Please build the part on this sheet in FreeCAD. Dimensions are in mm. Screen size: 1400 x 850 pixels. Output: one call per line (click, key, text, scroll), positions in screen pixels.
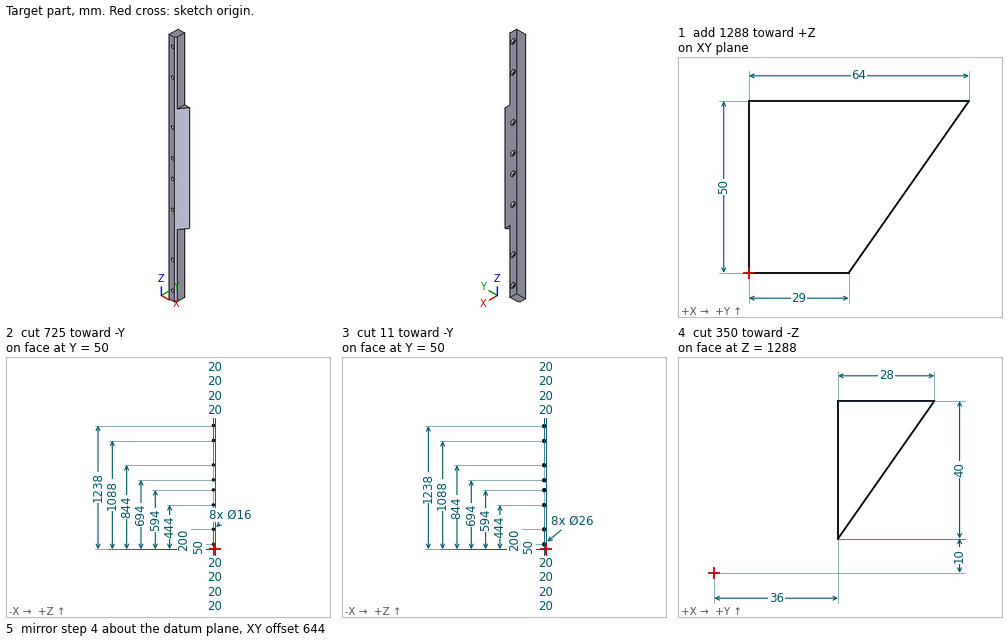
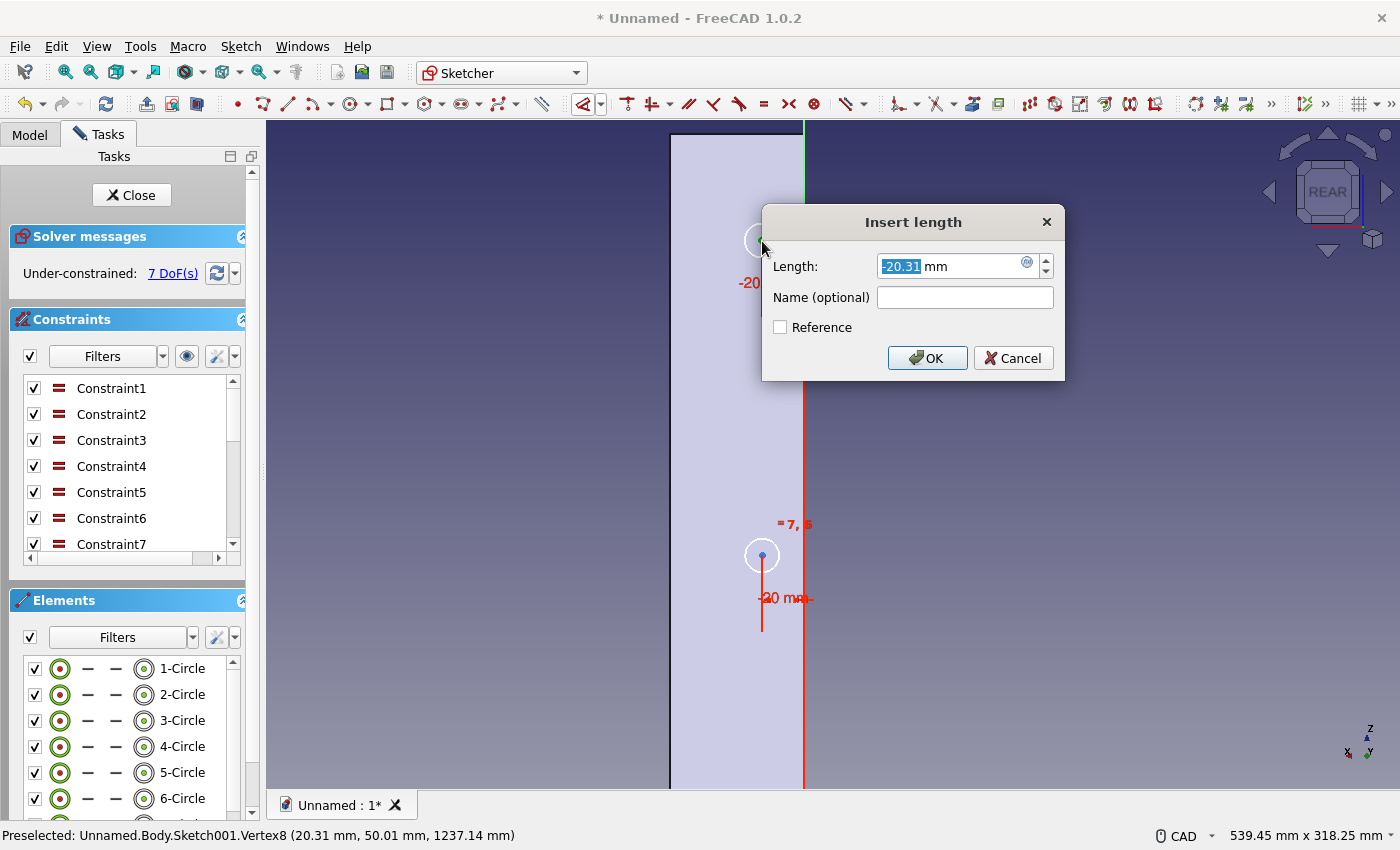
text(-20)
key(Return)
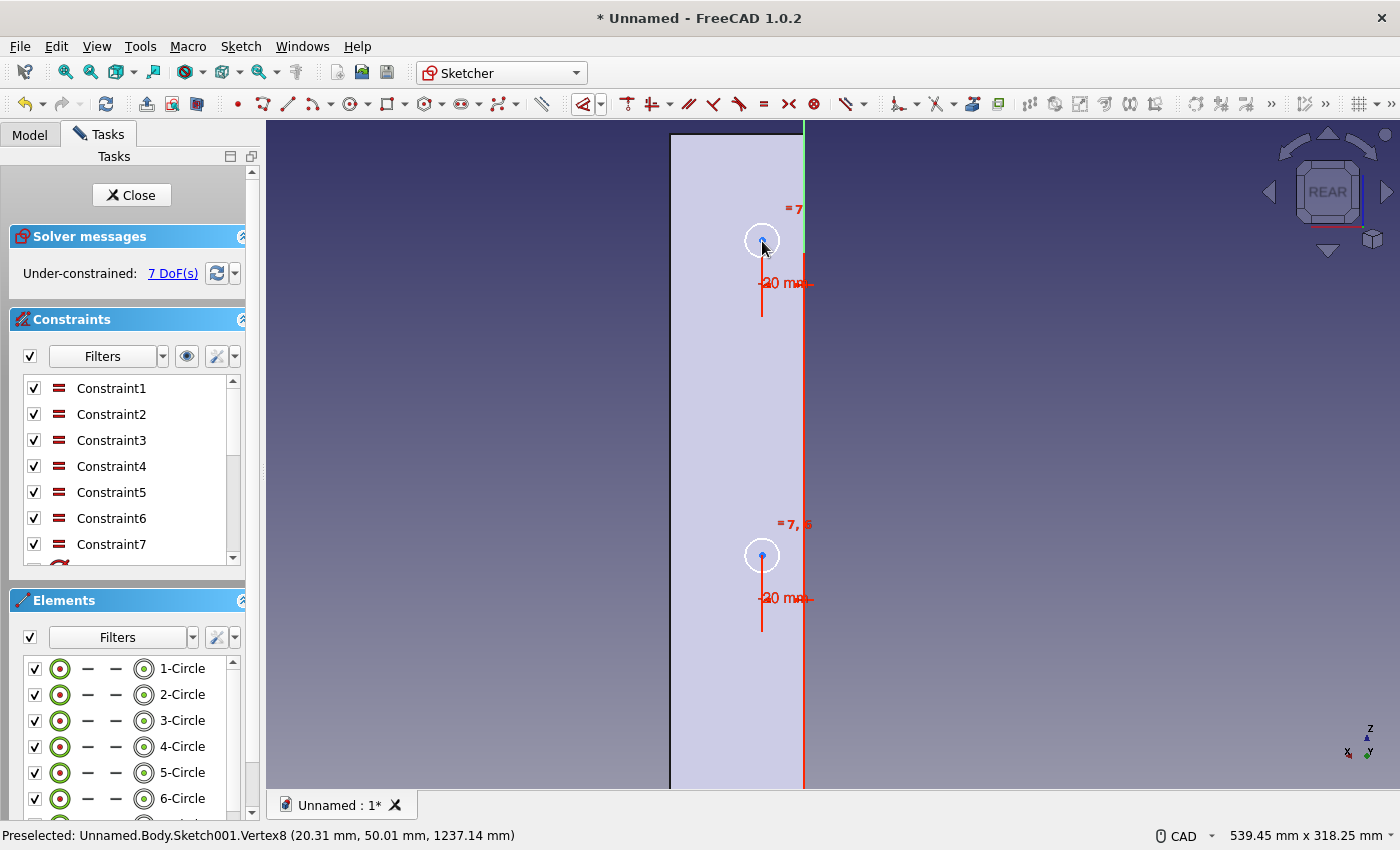
scroll(762, 241, down, 9)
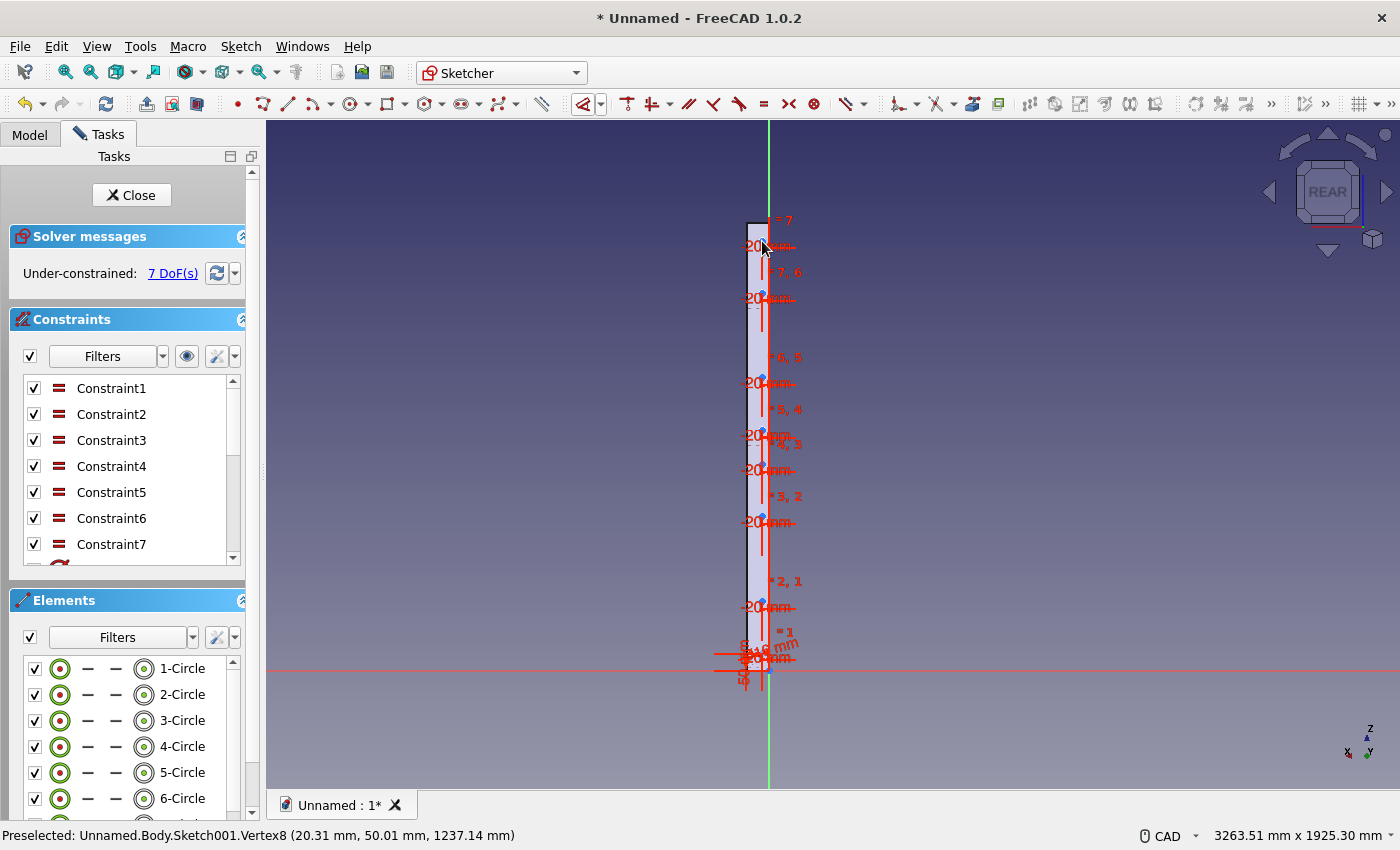
click(762, 602)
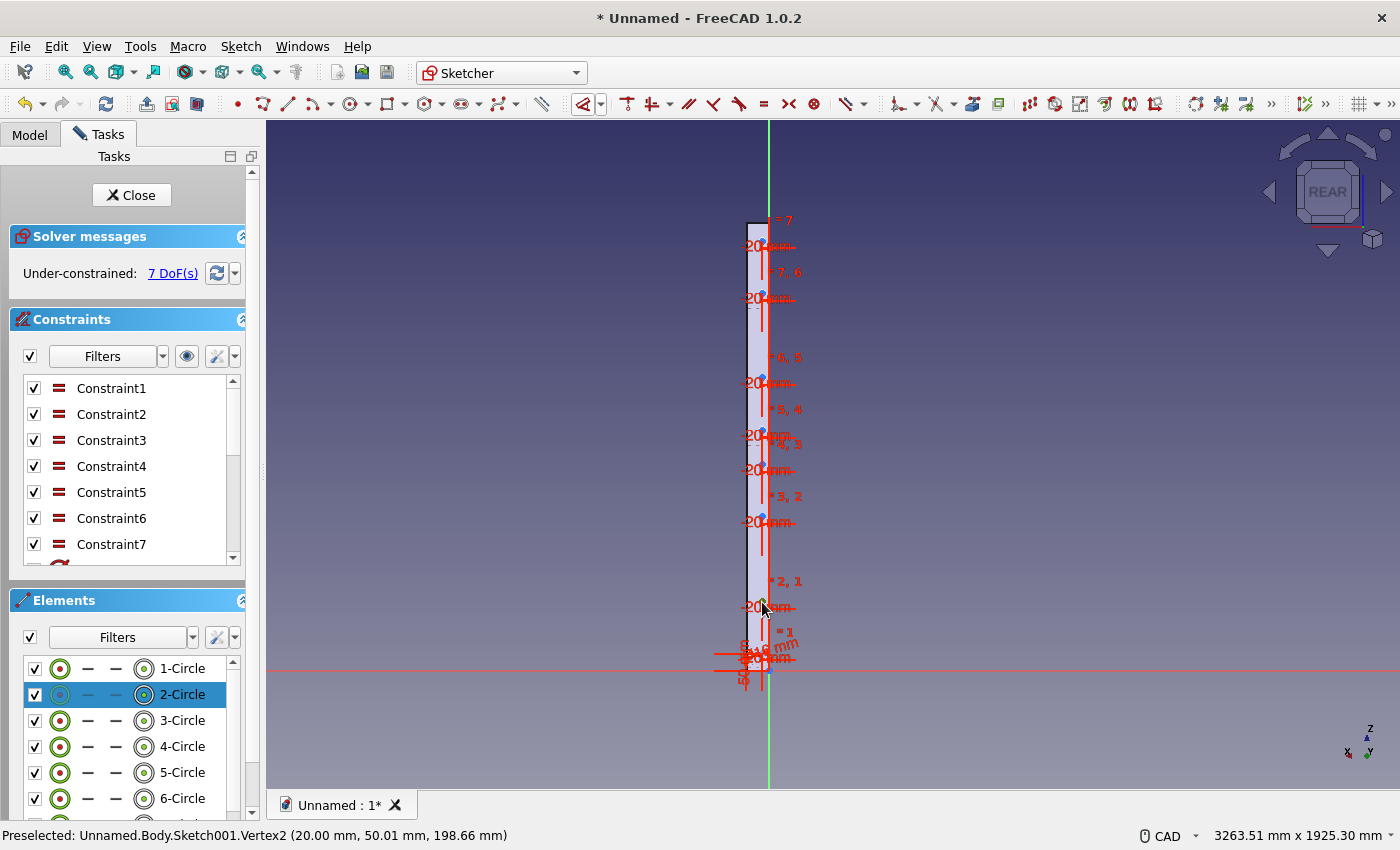
key(i)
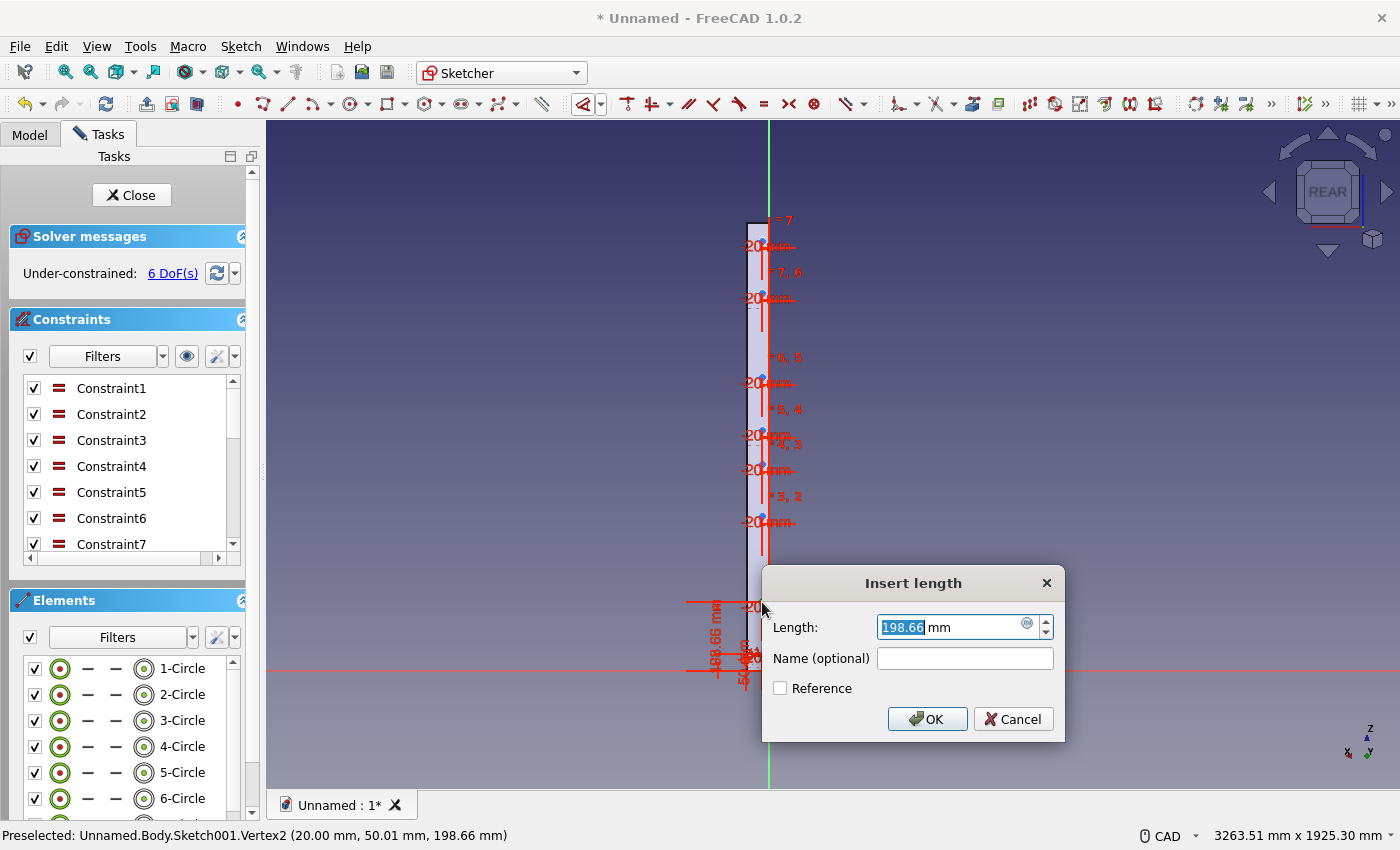
text(200)
key(Return)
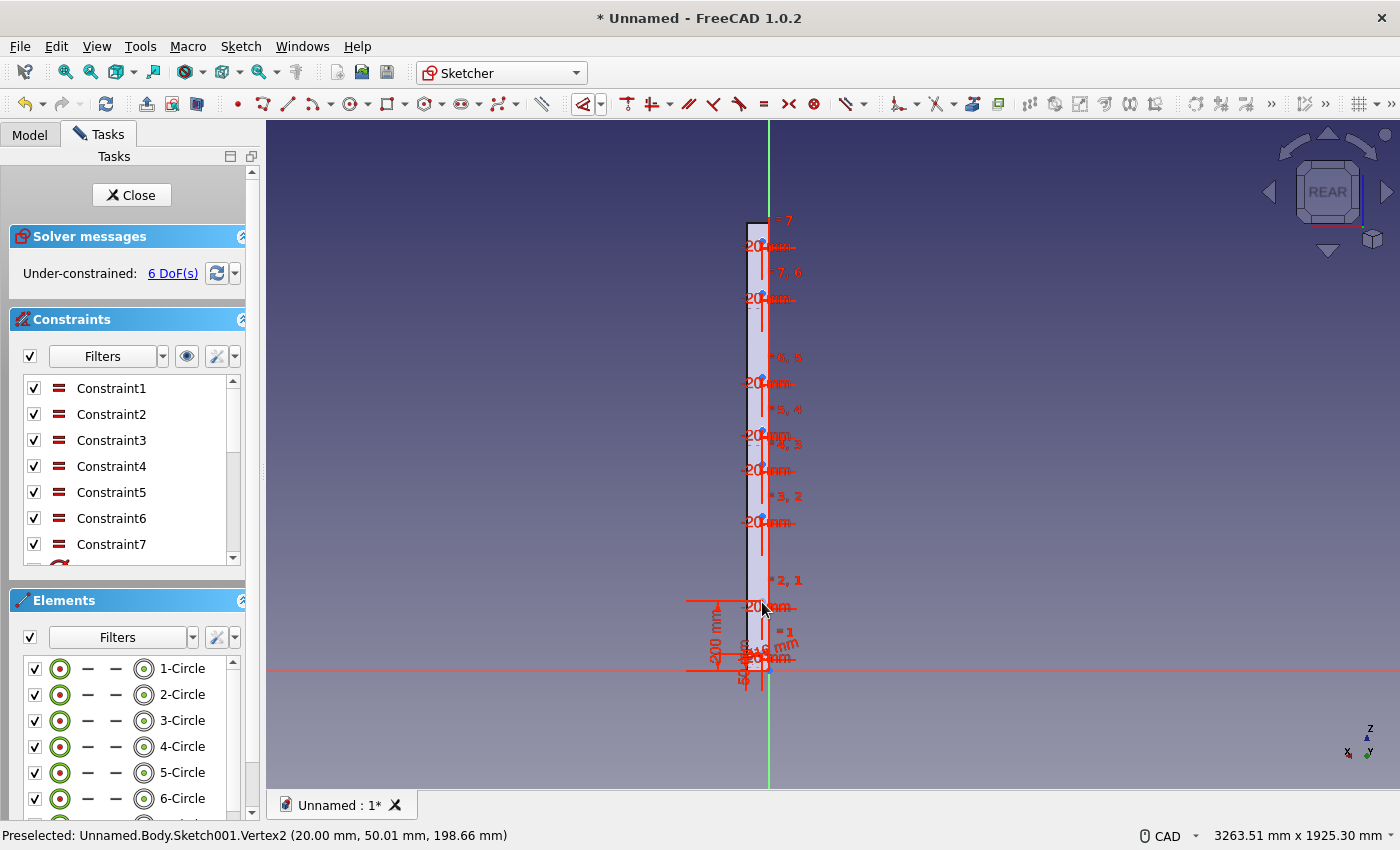
click(762, 517)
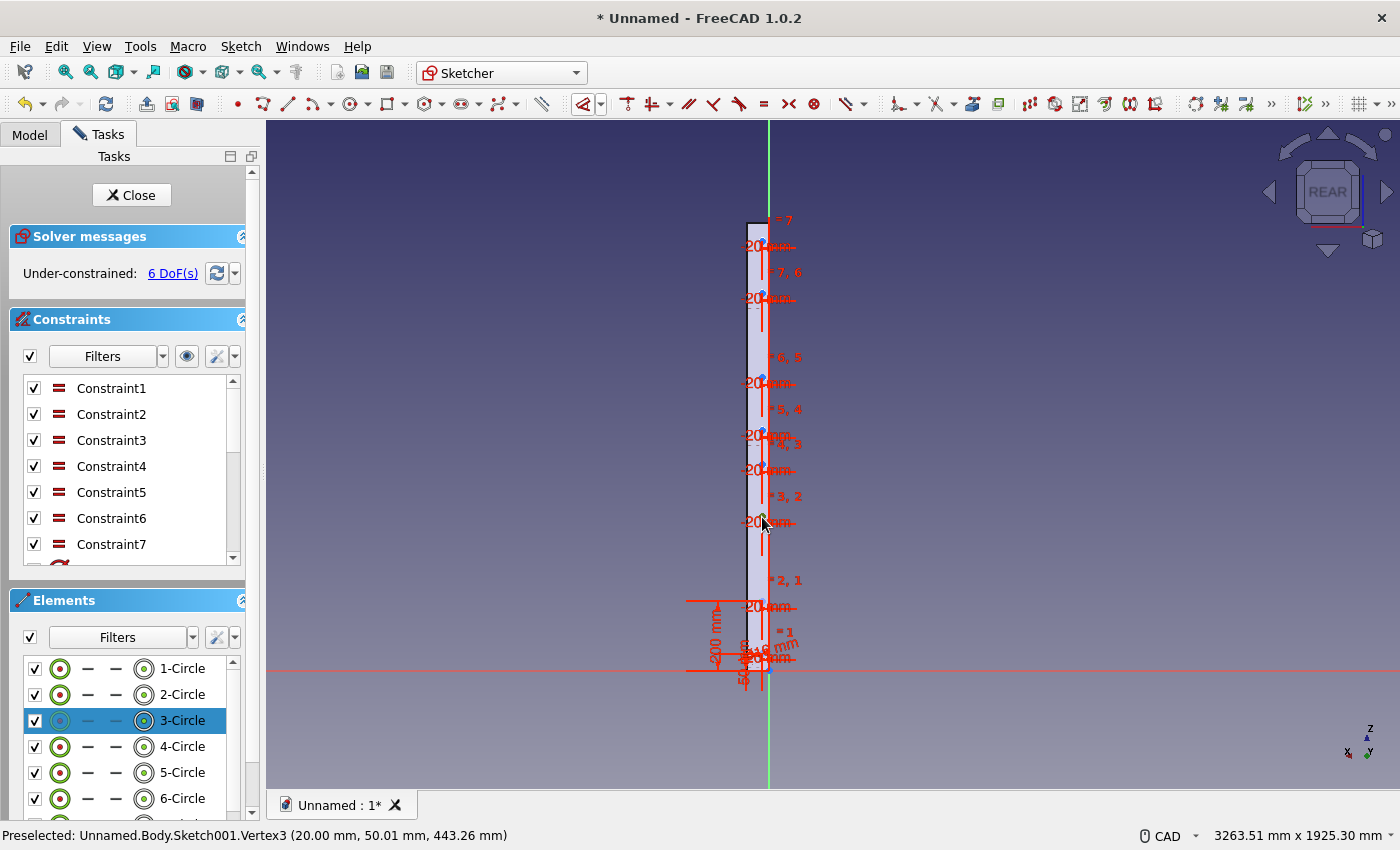
click(600, 104)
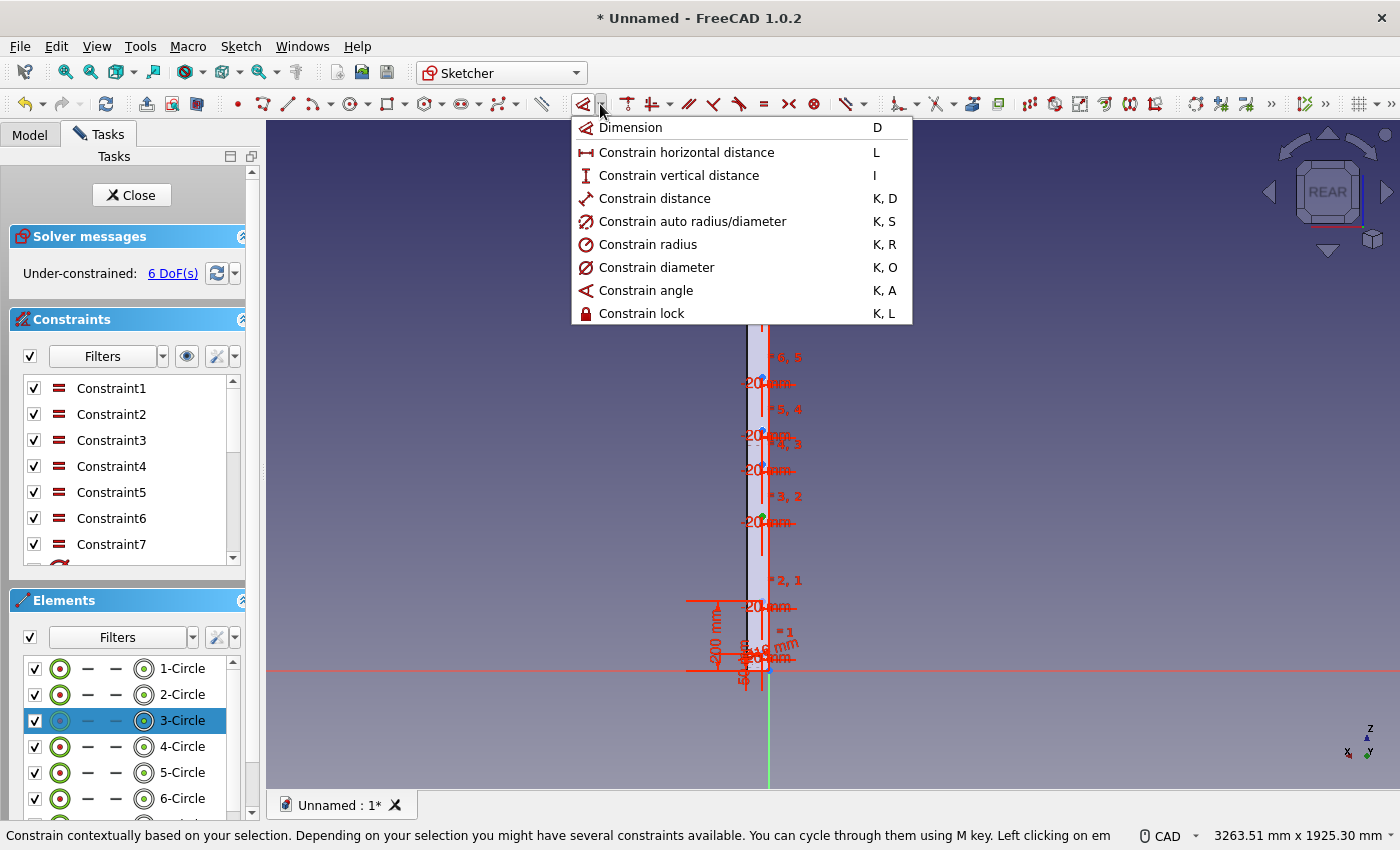
click(742, 176)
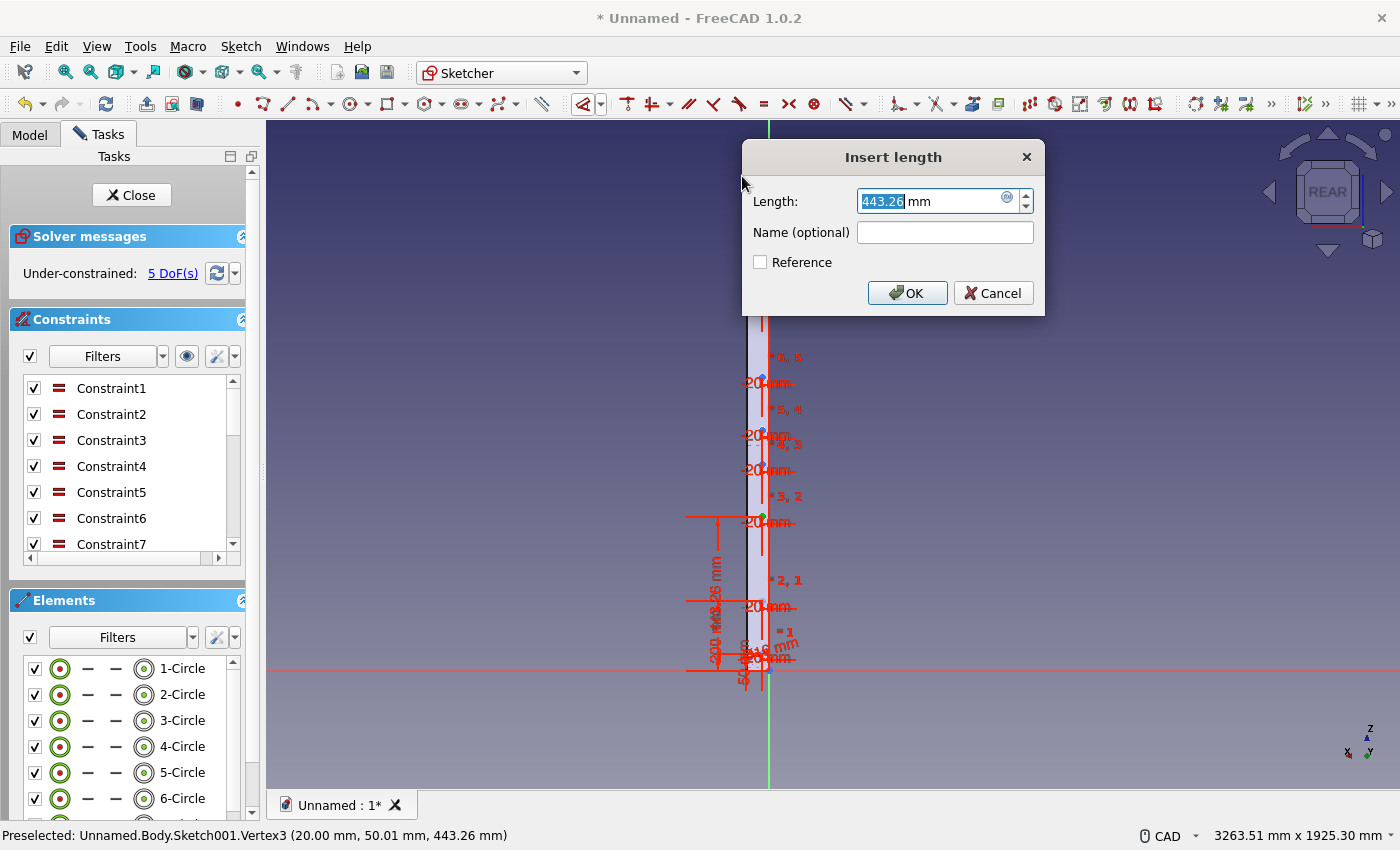
text(444)
key(Return)